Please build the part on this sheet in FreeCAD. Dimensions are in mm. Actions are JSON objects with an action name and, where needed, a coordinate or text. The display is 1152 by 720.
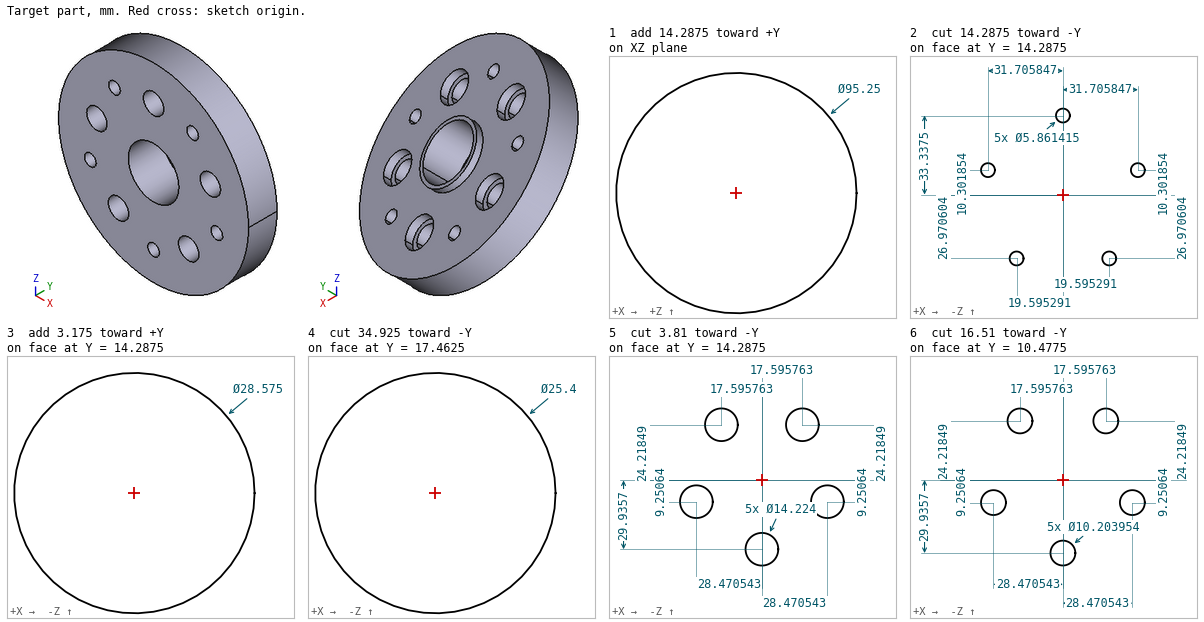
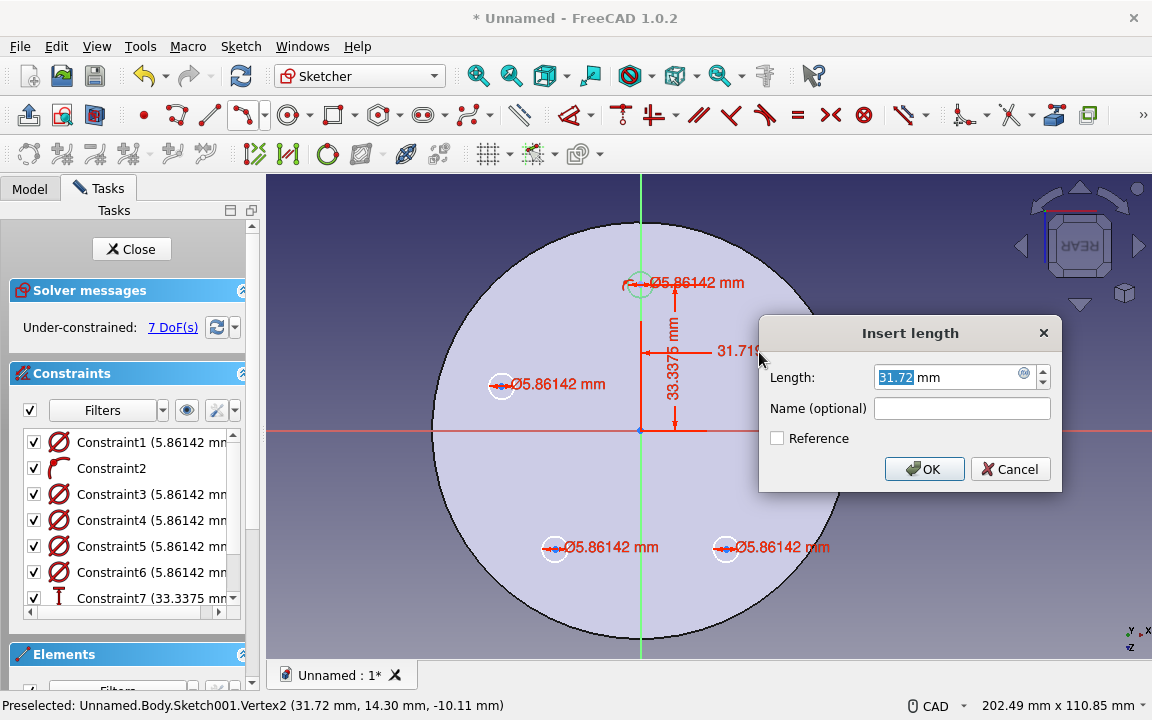
{"action": "type", "text": "31.705847"}
{"action": "key", "text": "Return"}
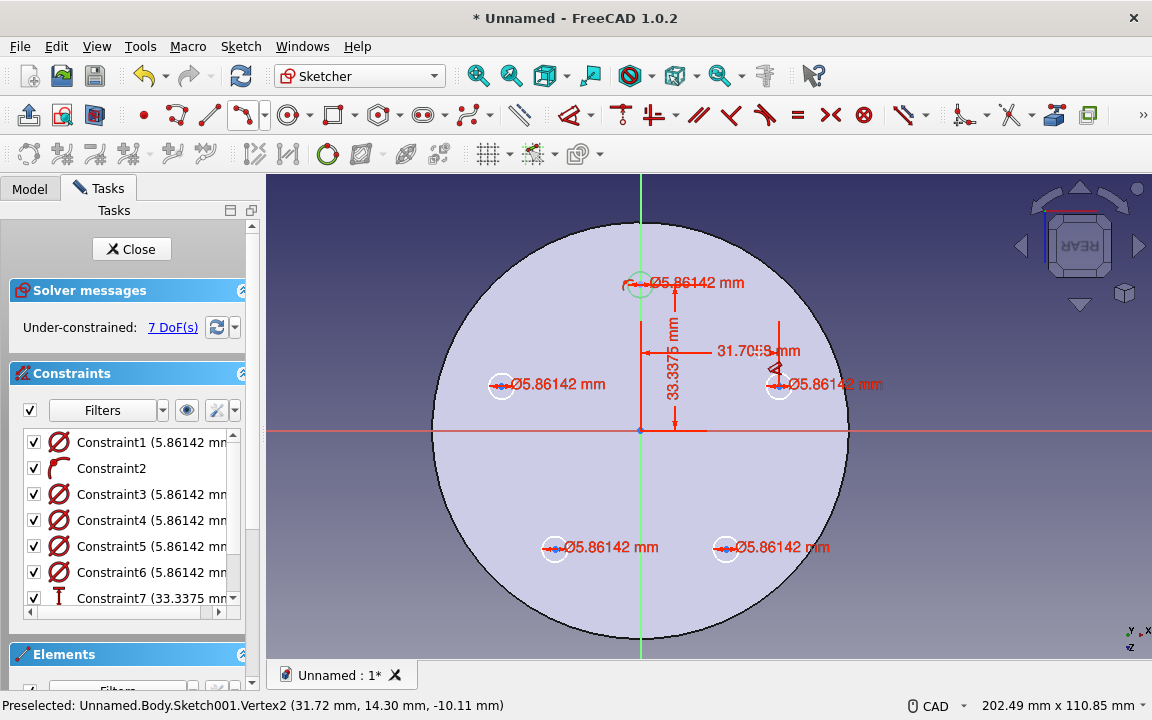
{"action": "left_click", "coordinate": [779, 386]}
{"action": "left_click", "coordinate": [813, 409]}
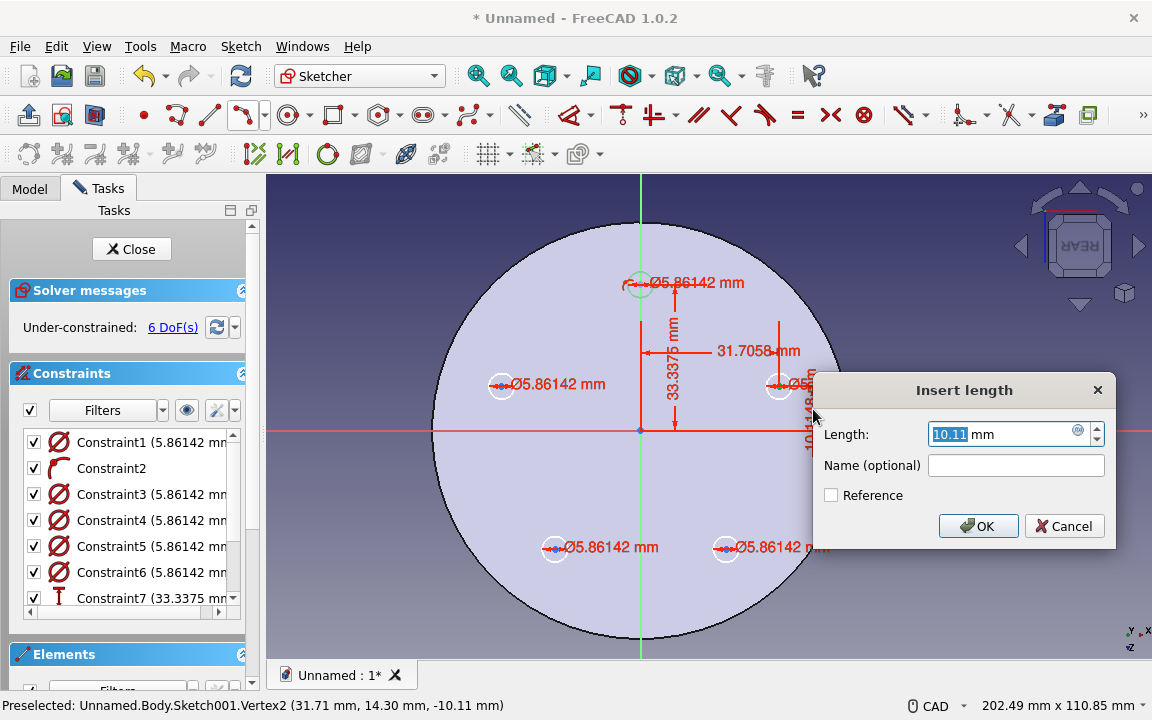
{"action": "type", "text": "10.301854"}
{"action": "key", "text": "Return"}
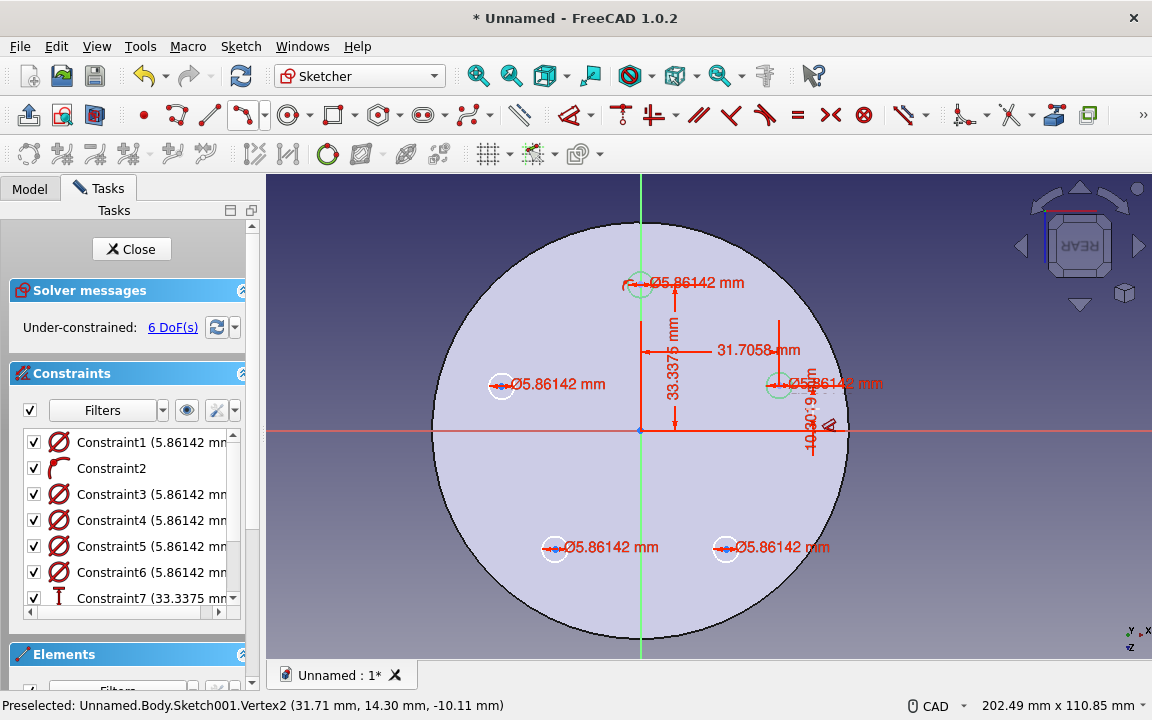
{"action": "left_click", "coordinate": [726, 549]}
{"action": "left_click", "coordinate": [683, 583]}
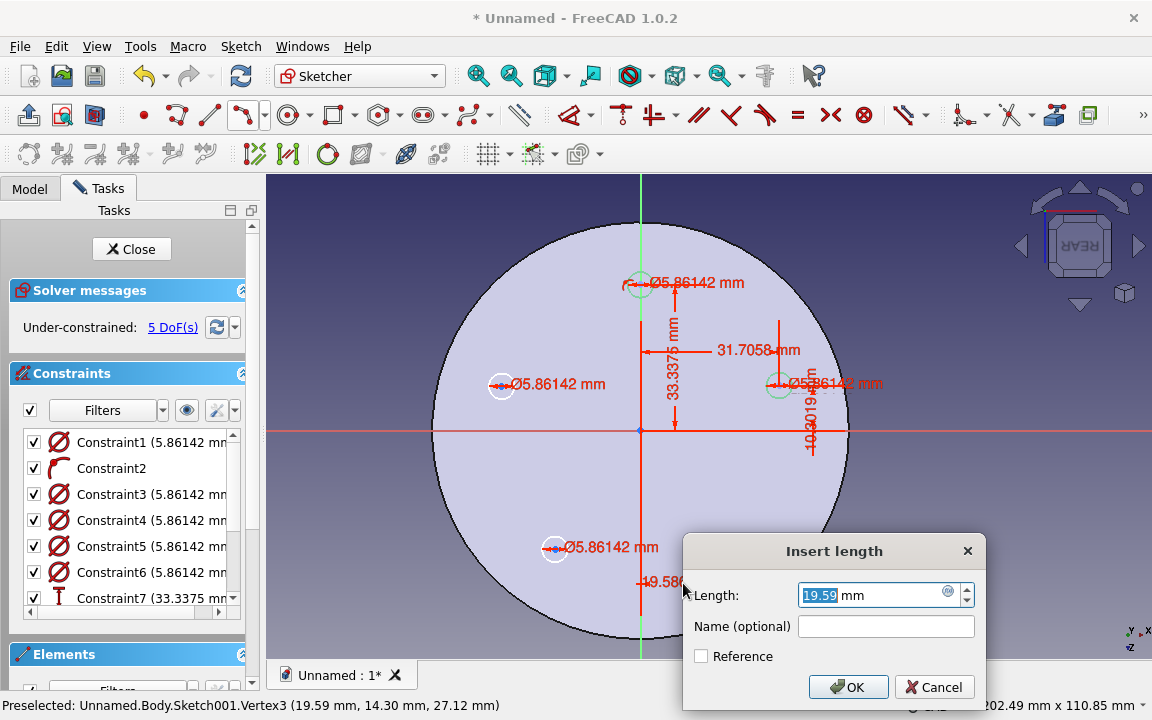
{"action": "type", "text": "19.595291"}
{"action": "key", "text": "Return"}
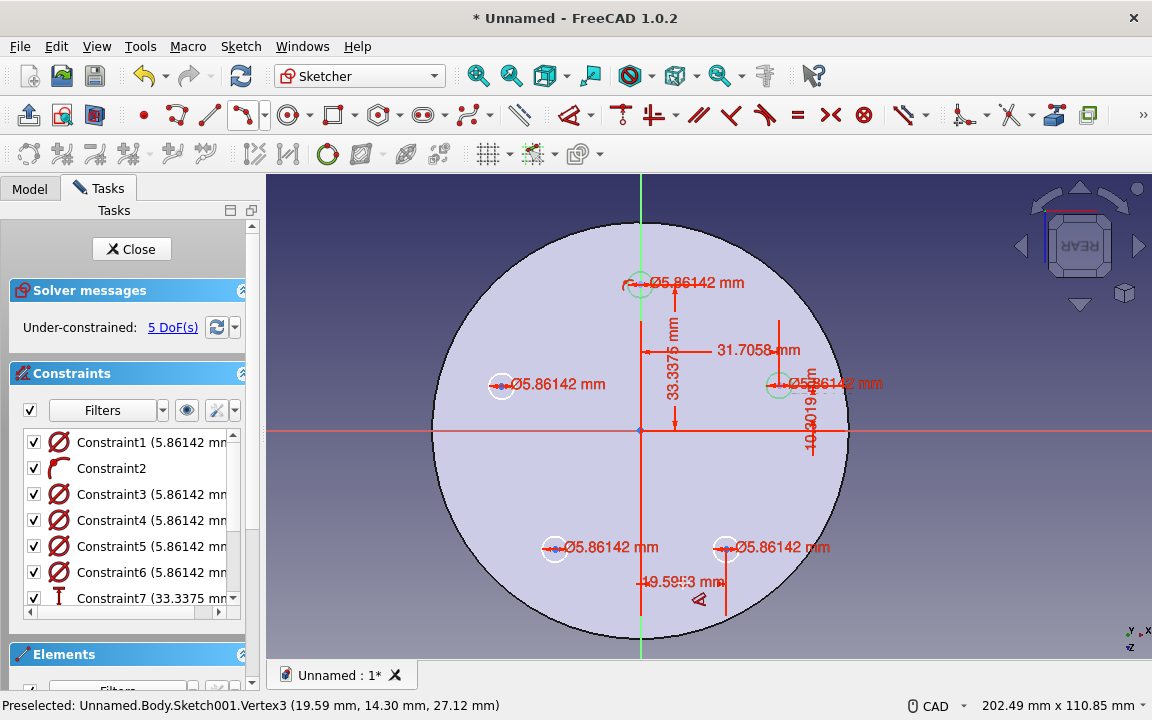
{"action": "left_click", "coordinate": [726, 549]}
{"action": "left_click", "coordinate": [760, 490]}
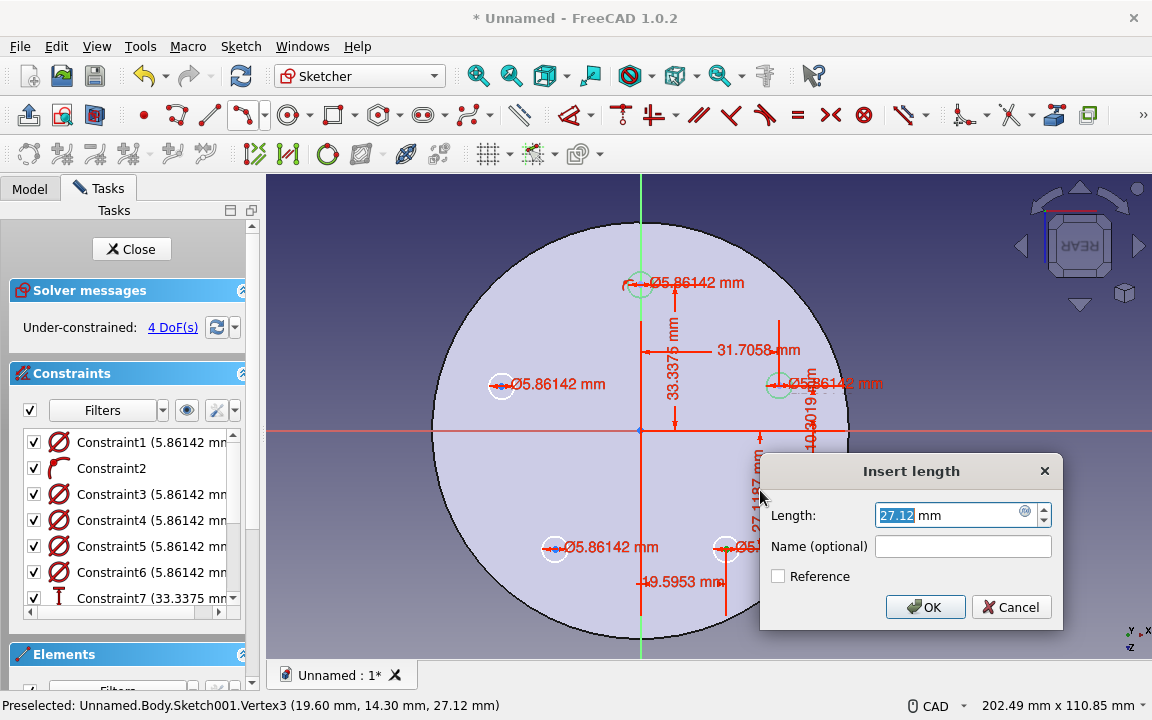
{"action": "type", "text": "26.970604"}
{"action": "key", "text": "Return"}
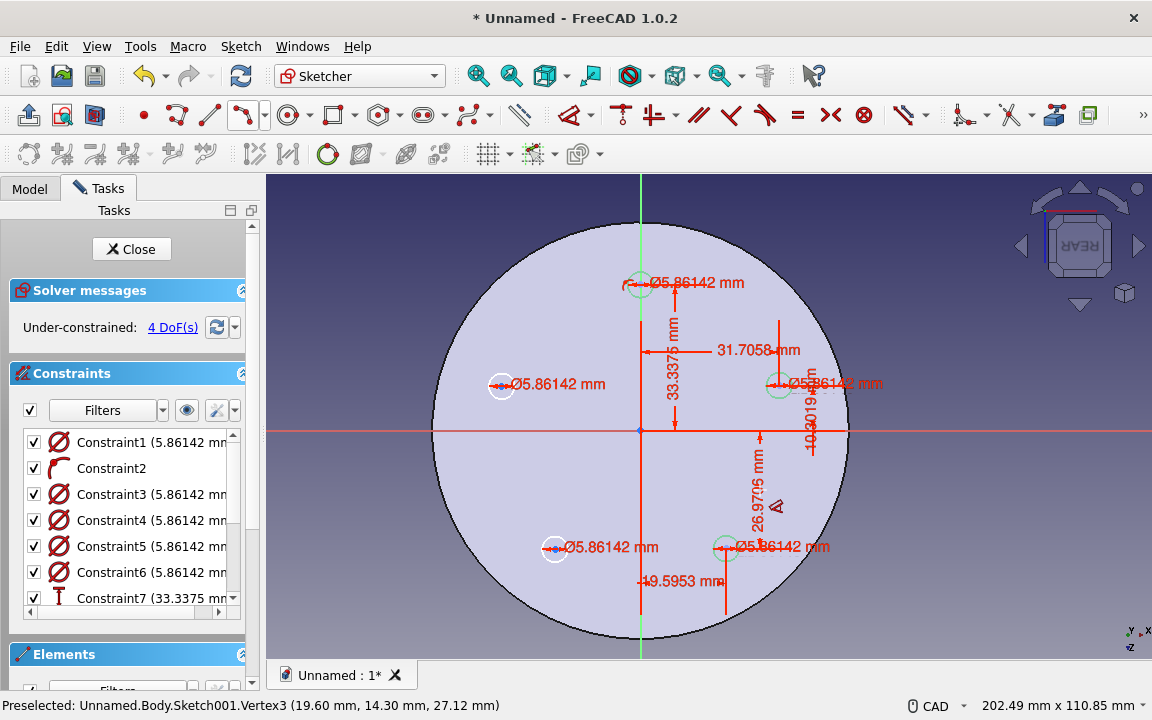
{"action": "left_click", "coordinate": [555, 549]}
{"action": "left_click", "coordinate": [598, 583]}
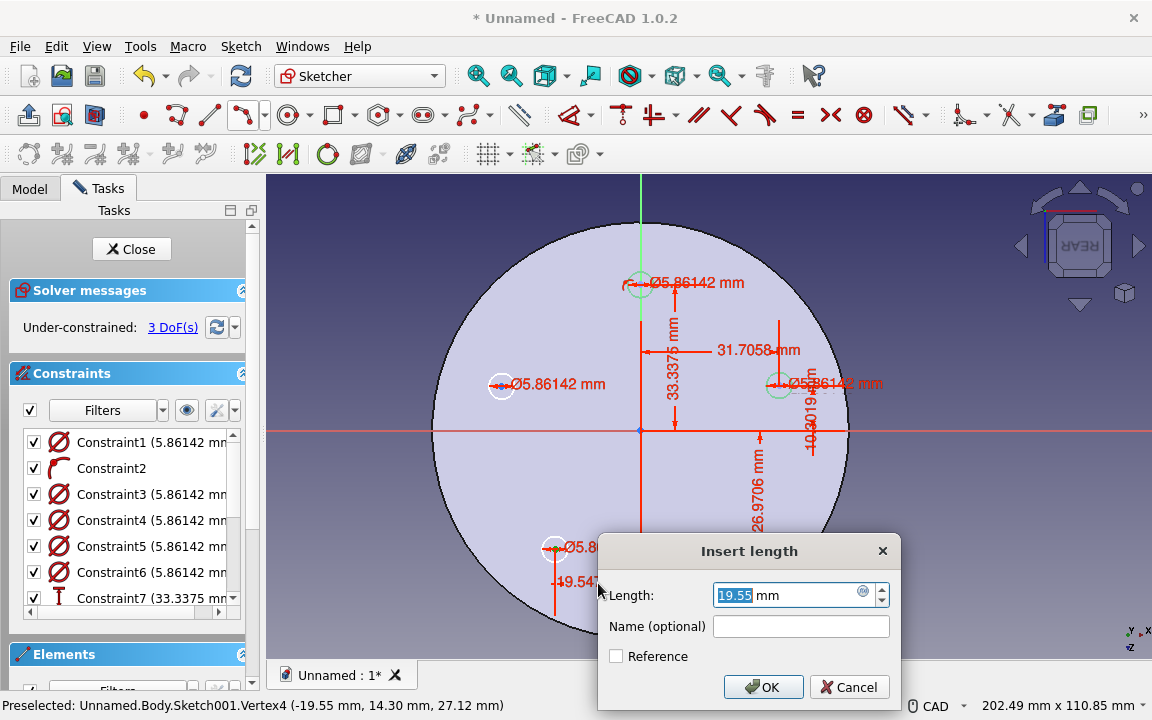
{"action": "type", "text": "19.595291"}
{"action": "key", "text": "Return"}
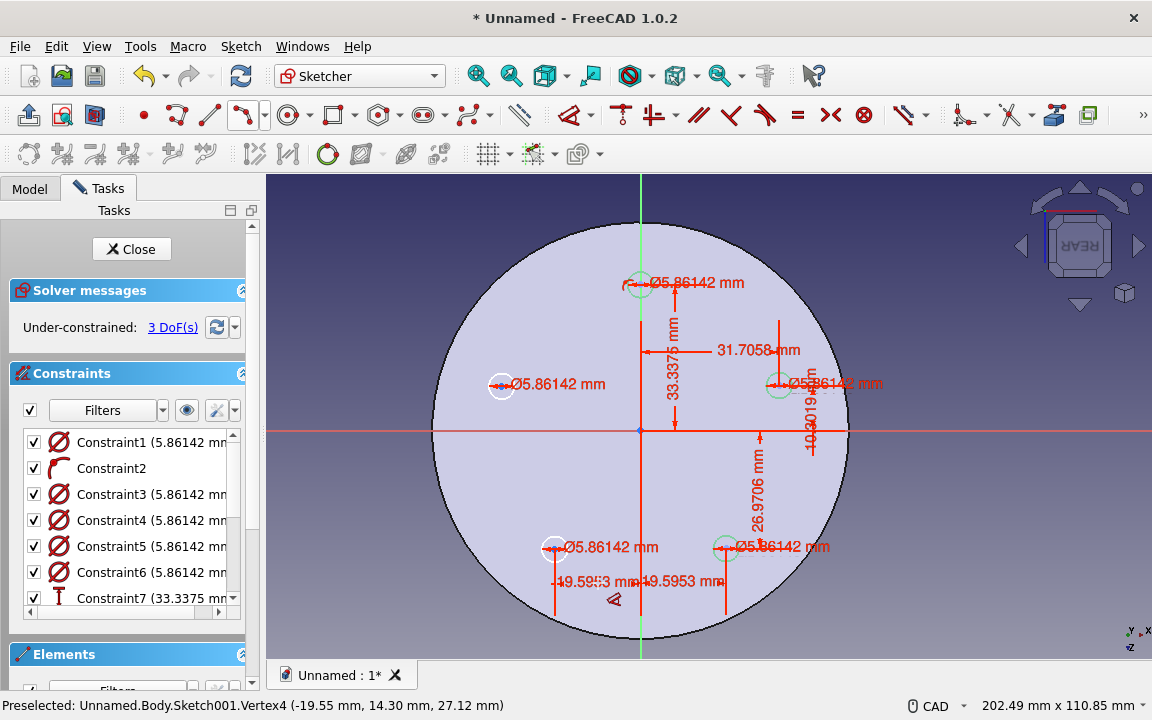
{"action": "left_click", "coordinate": [555, 549]}
{"action": "left_click", "coordinate": [521, 490]}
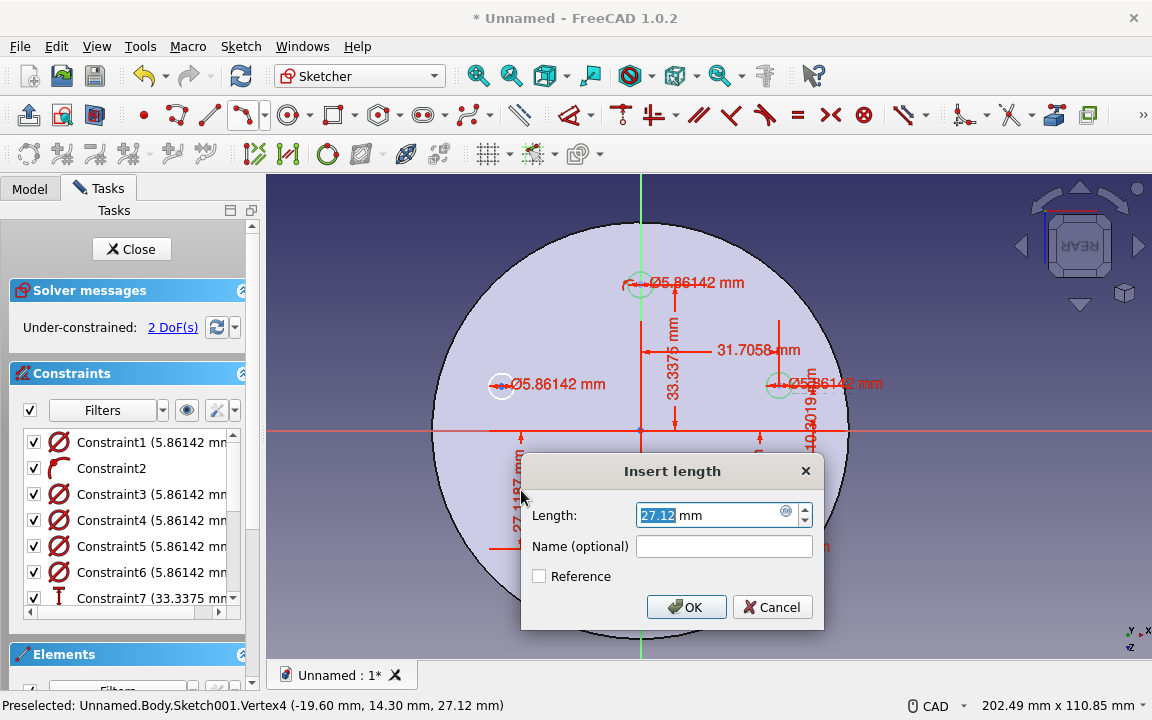
{"action": "type", "text": "26.970604"}
{"action": "key", "text": "Return"}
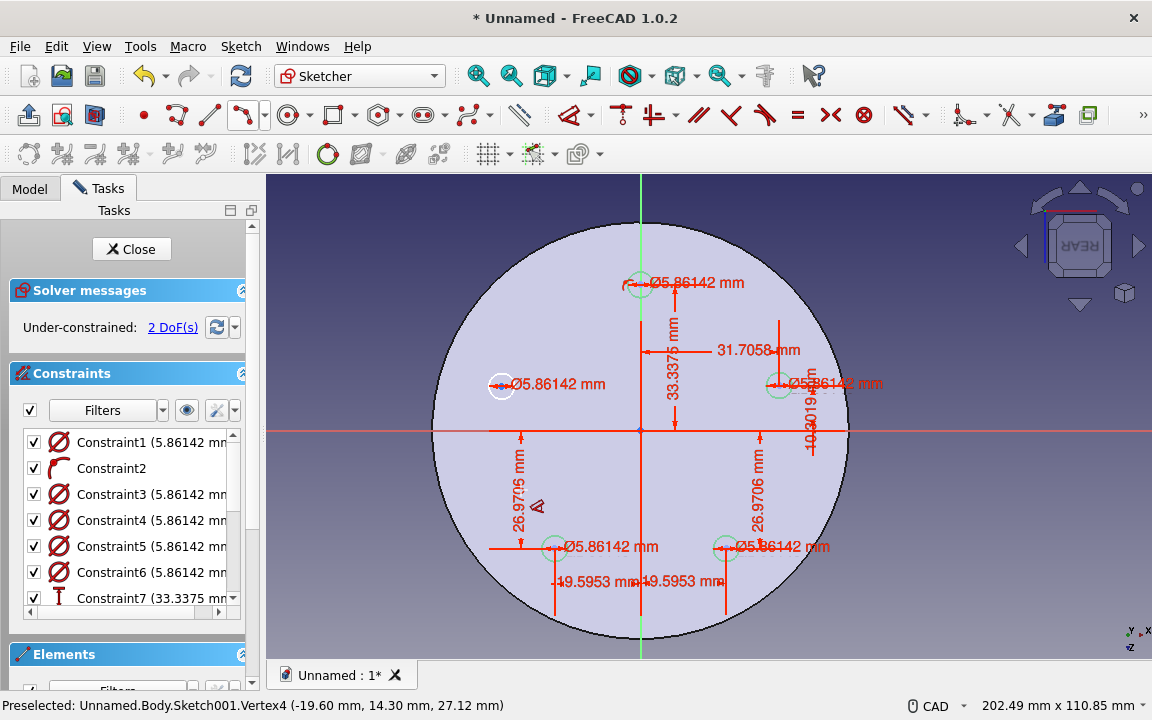
{"action": "left_click", "coordinate": [502, 386]}
{"action": "left_click", "coordinate": [571, 352]}